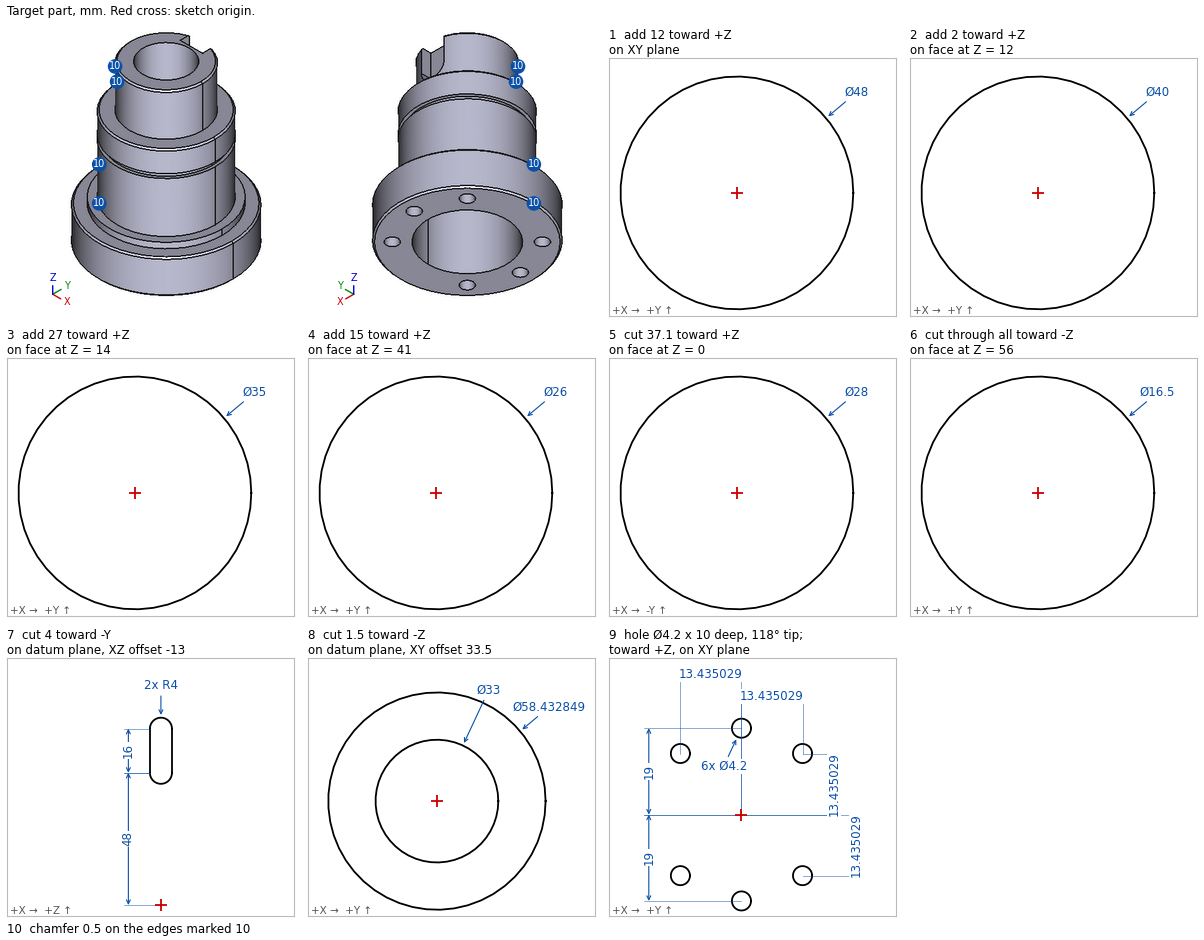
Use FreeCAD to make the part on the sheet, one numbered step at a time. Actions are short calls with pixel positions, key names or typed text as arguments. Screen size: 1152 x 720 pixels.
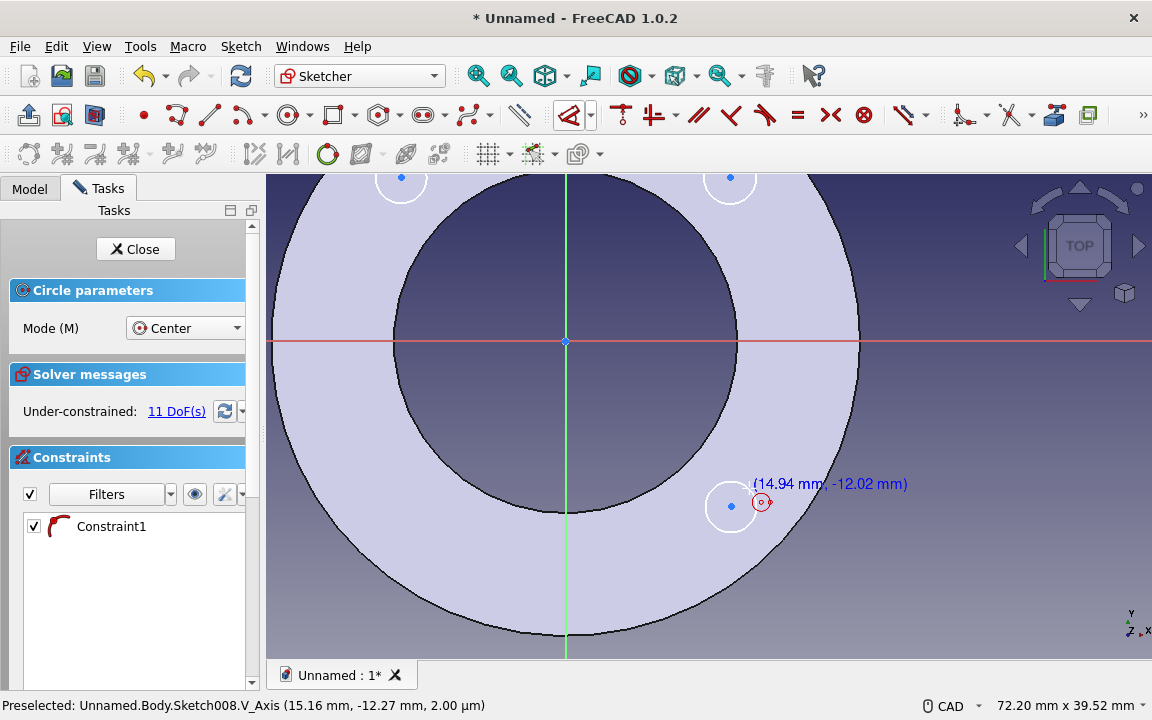
click(566, 575)
click(584, 556)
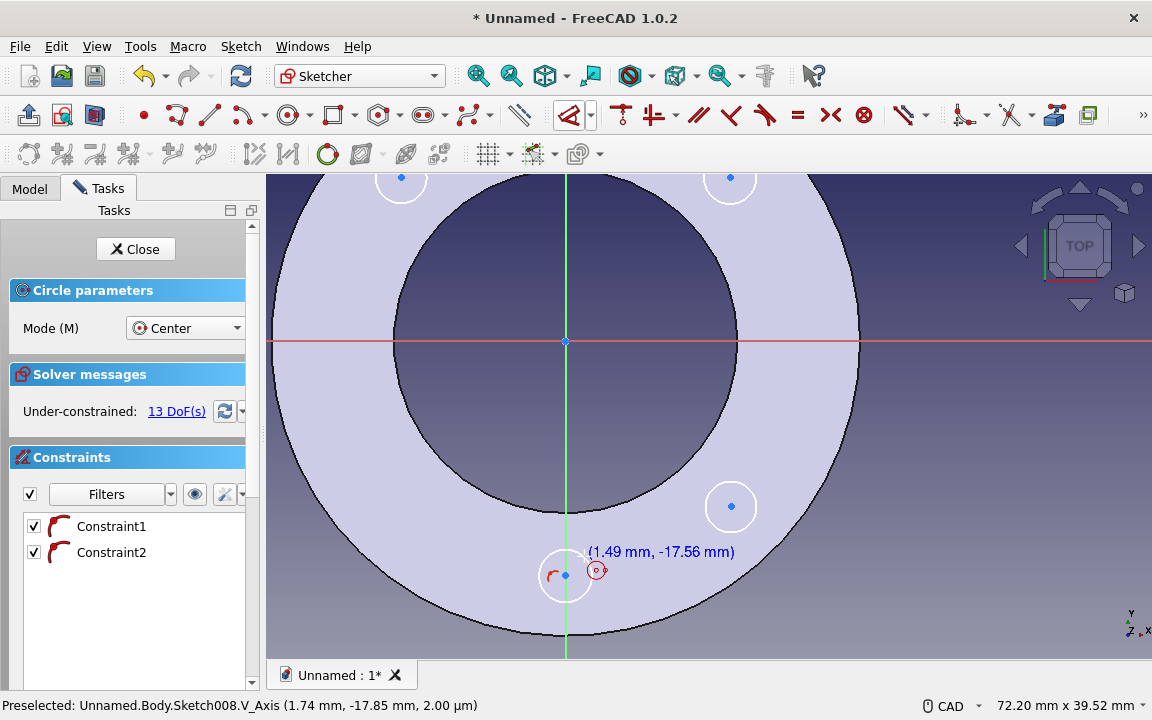
click(401, 506)
click(419, 488)
key(Escape)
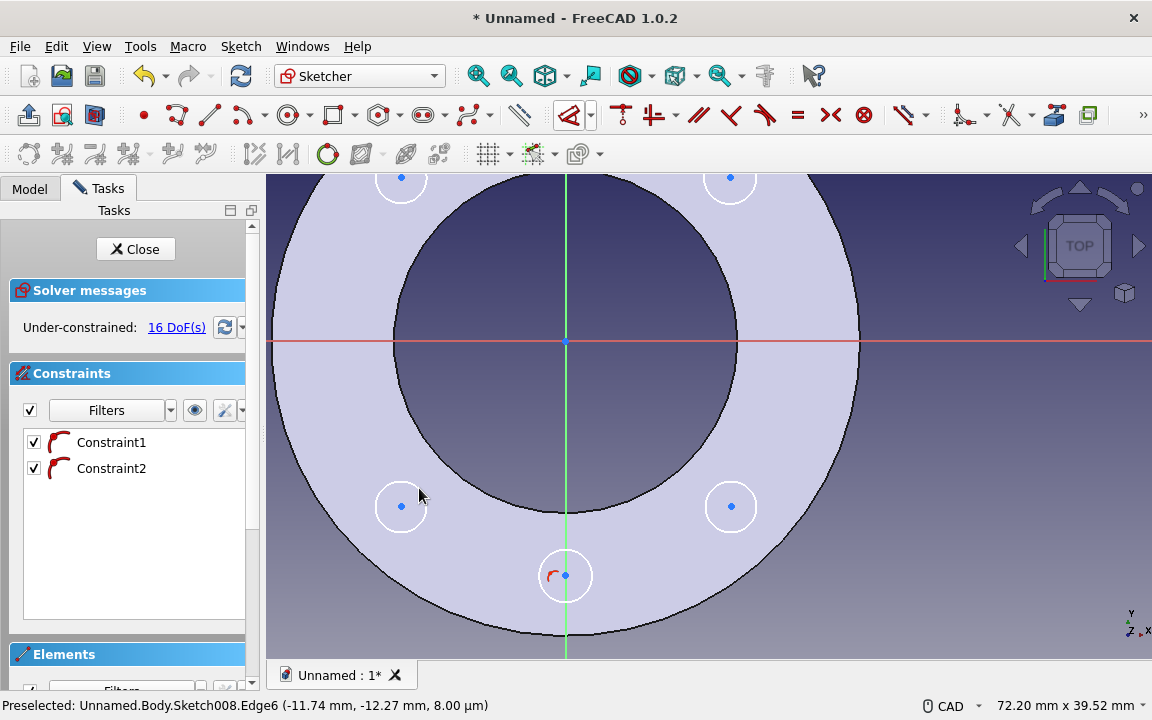
scroll(732, 508, down, 3)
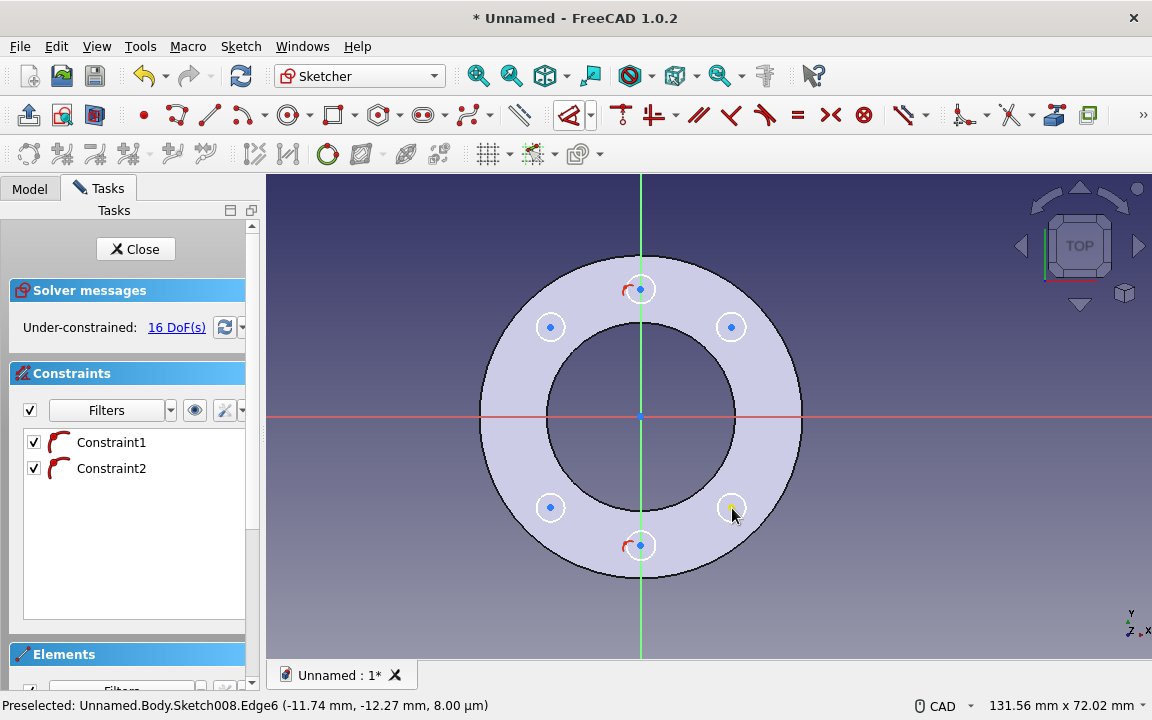
scroll(651, 279, up, 2)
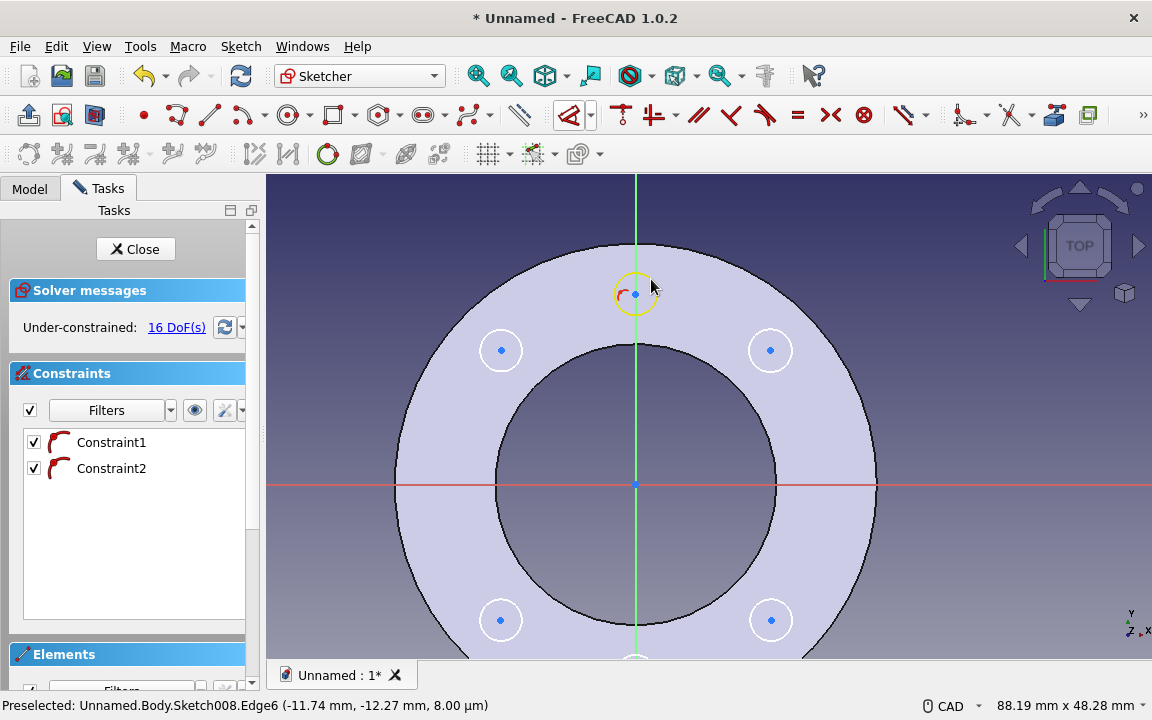
click(651, 279)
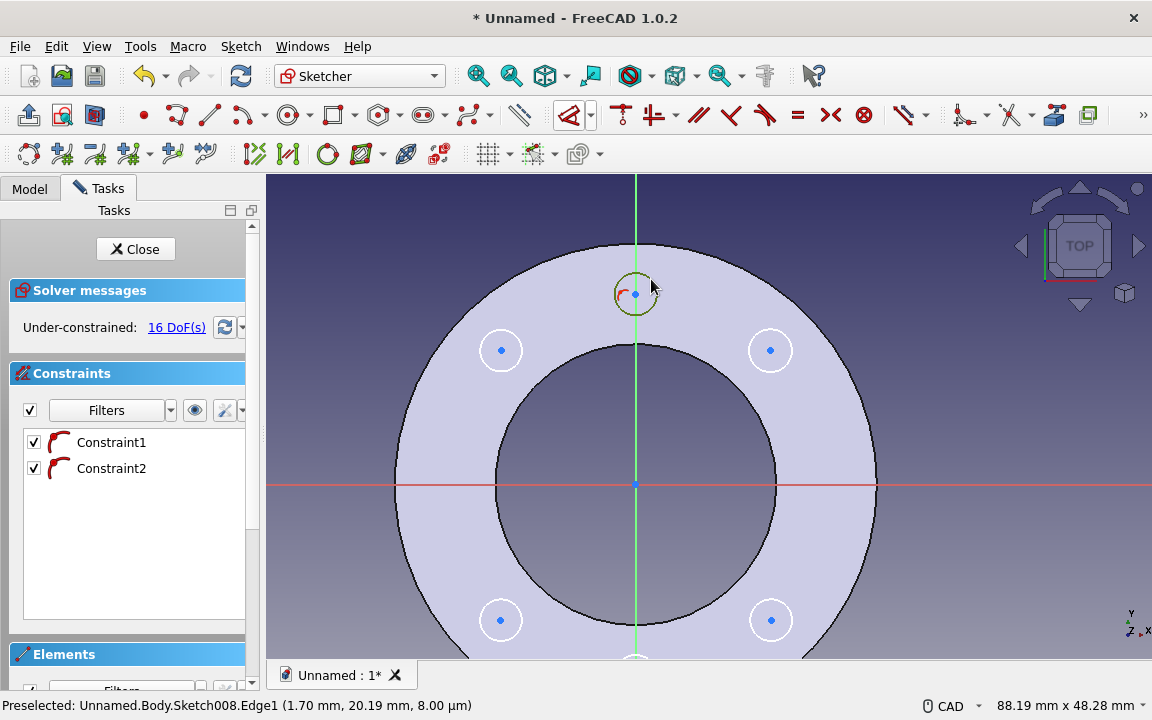
click(786, 335)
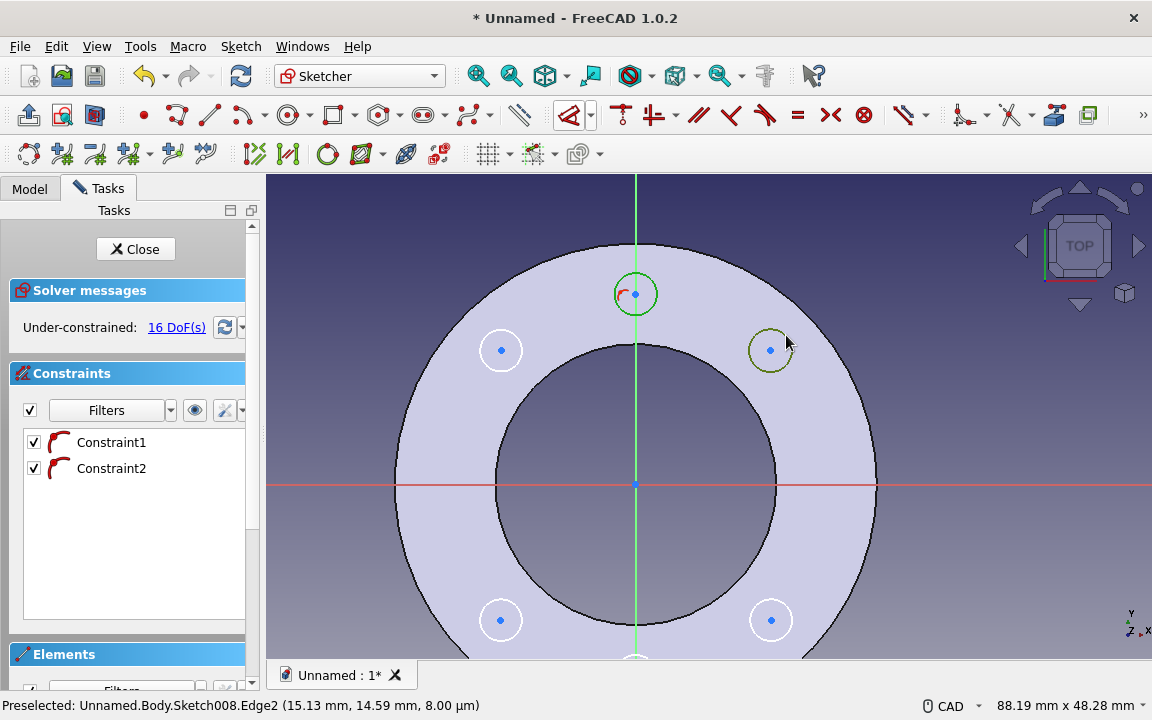
click(516, 336)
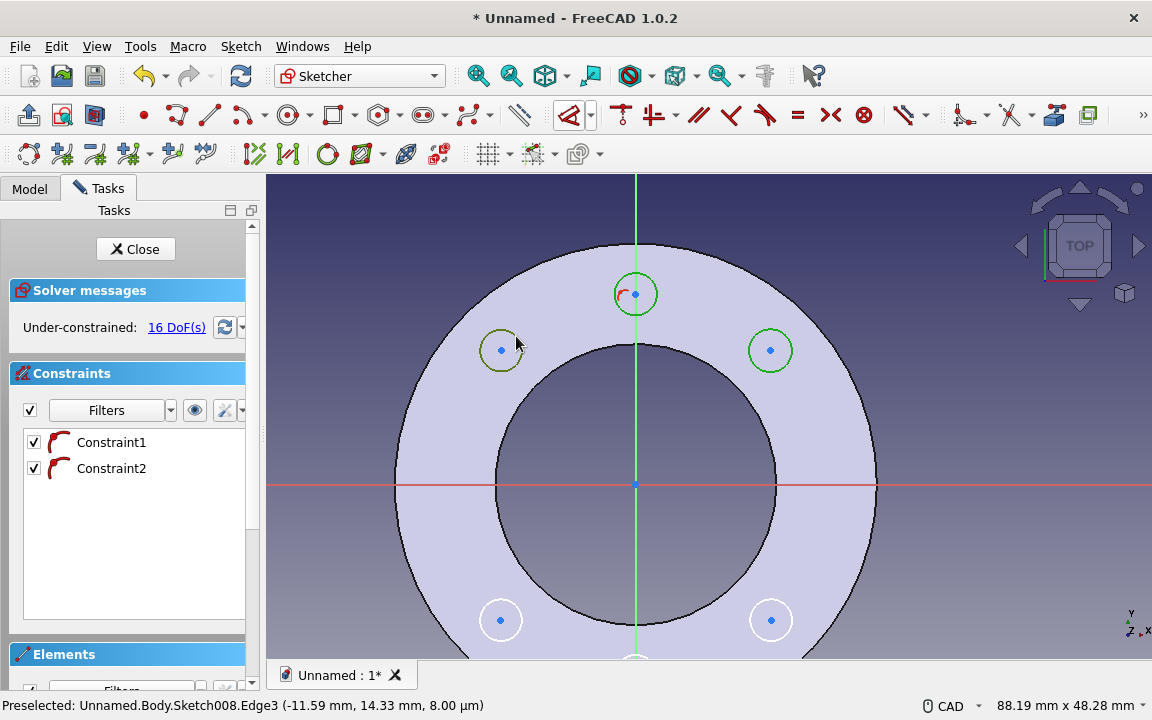
click(786, 605)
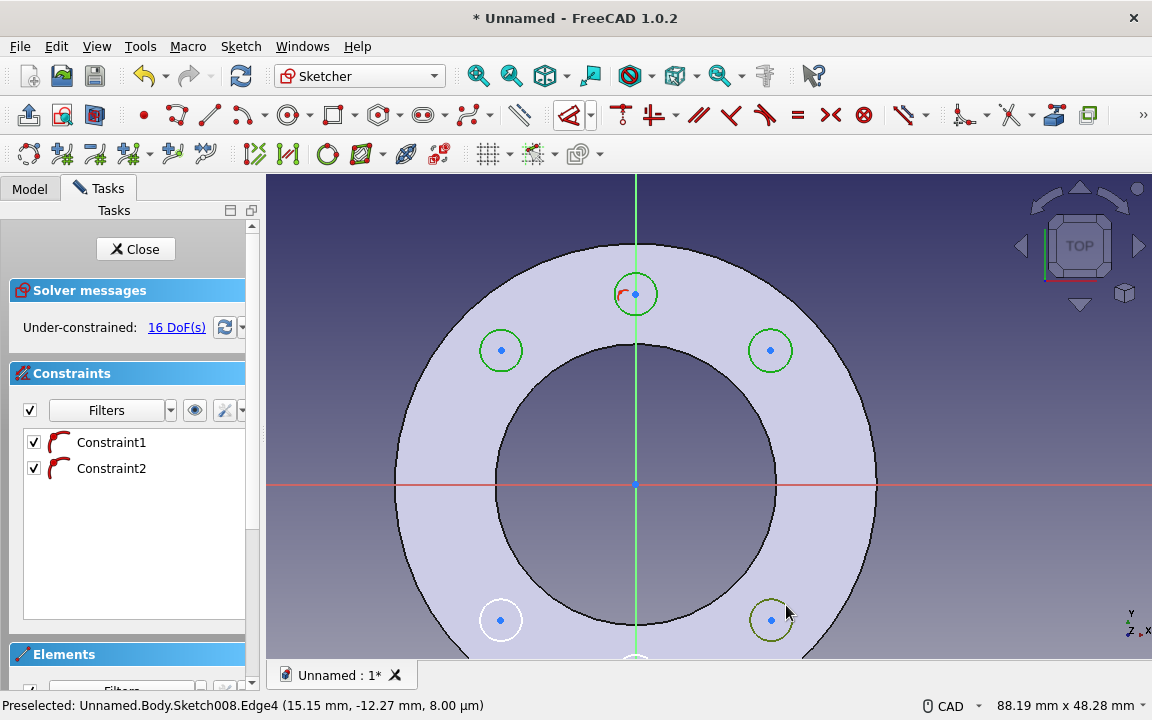
scroll(650, 278, down, 2)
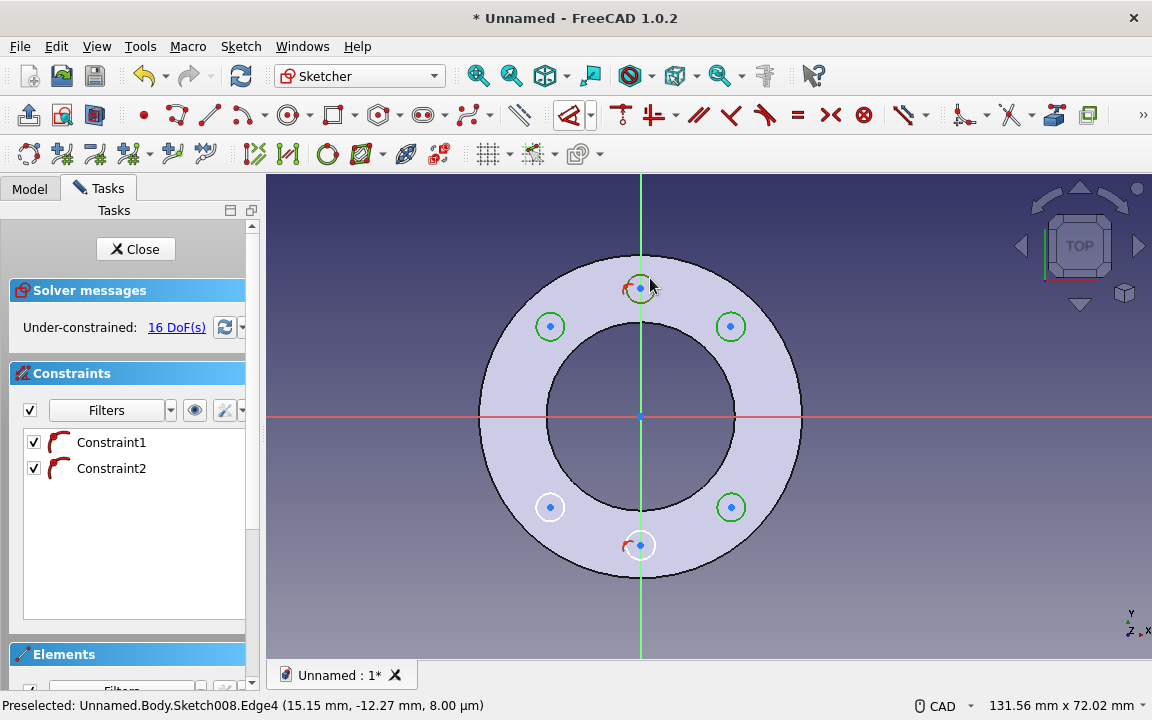
scroll(651, 535, up, 2)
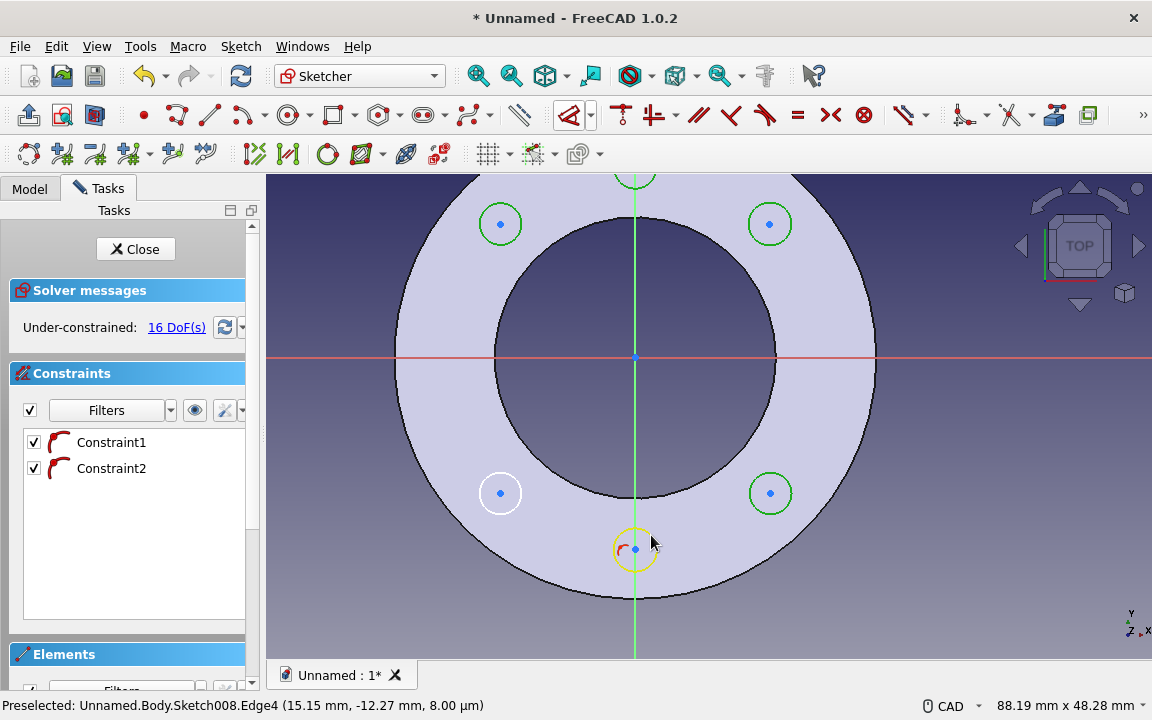
click(651, 535)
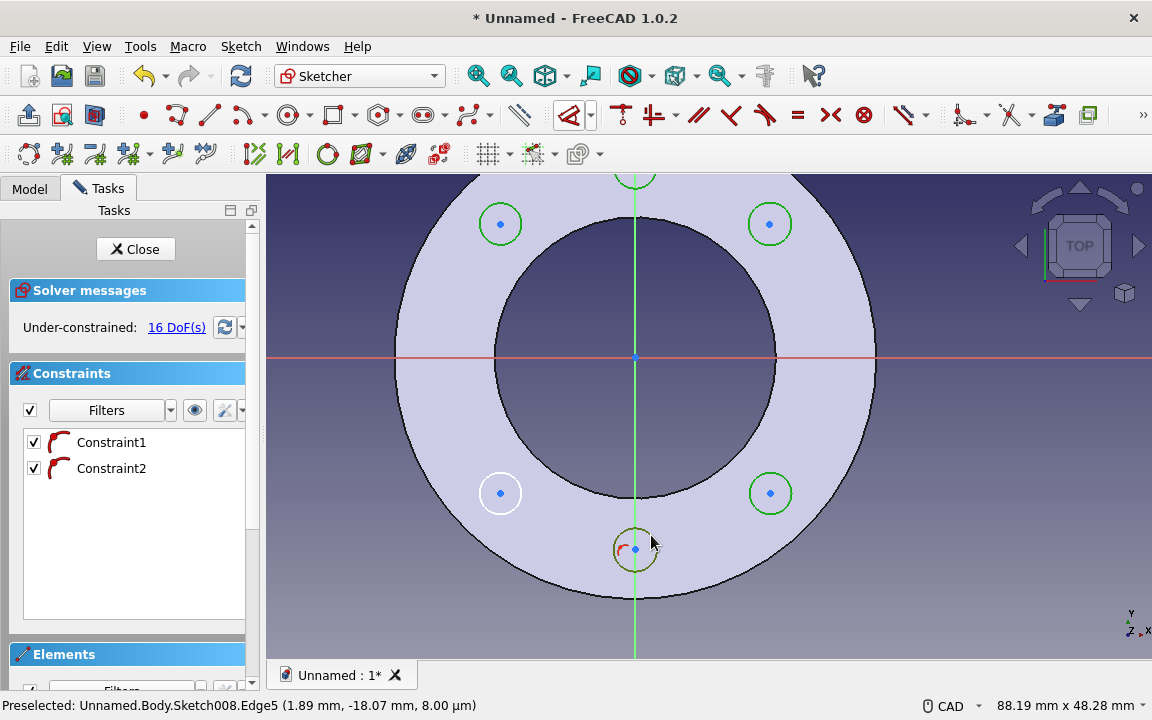
click(515, 479)